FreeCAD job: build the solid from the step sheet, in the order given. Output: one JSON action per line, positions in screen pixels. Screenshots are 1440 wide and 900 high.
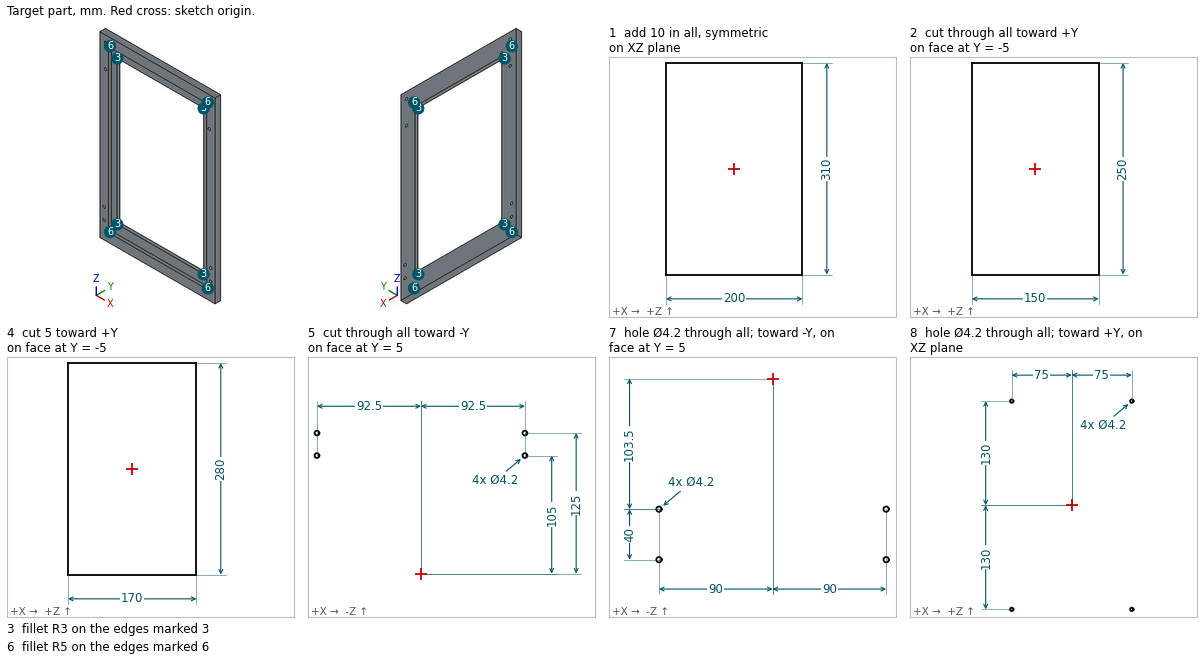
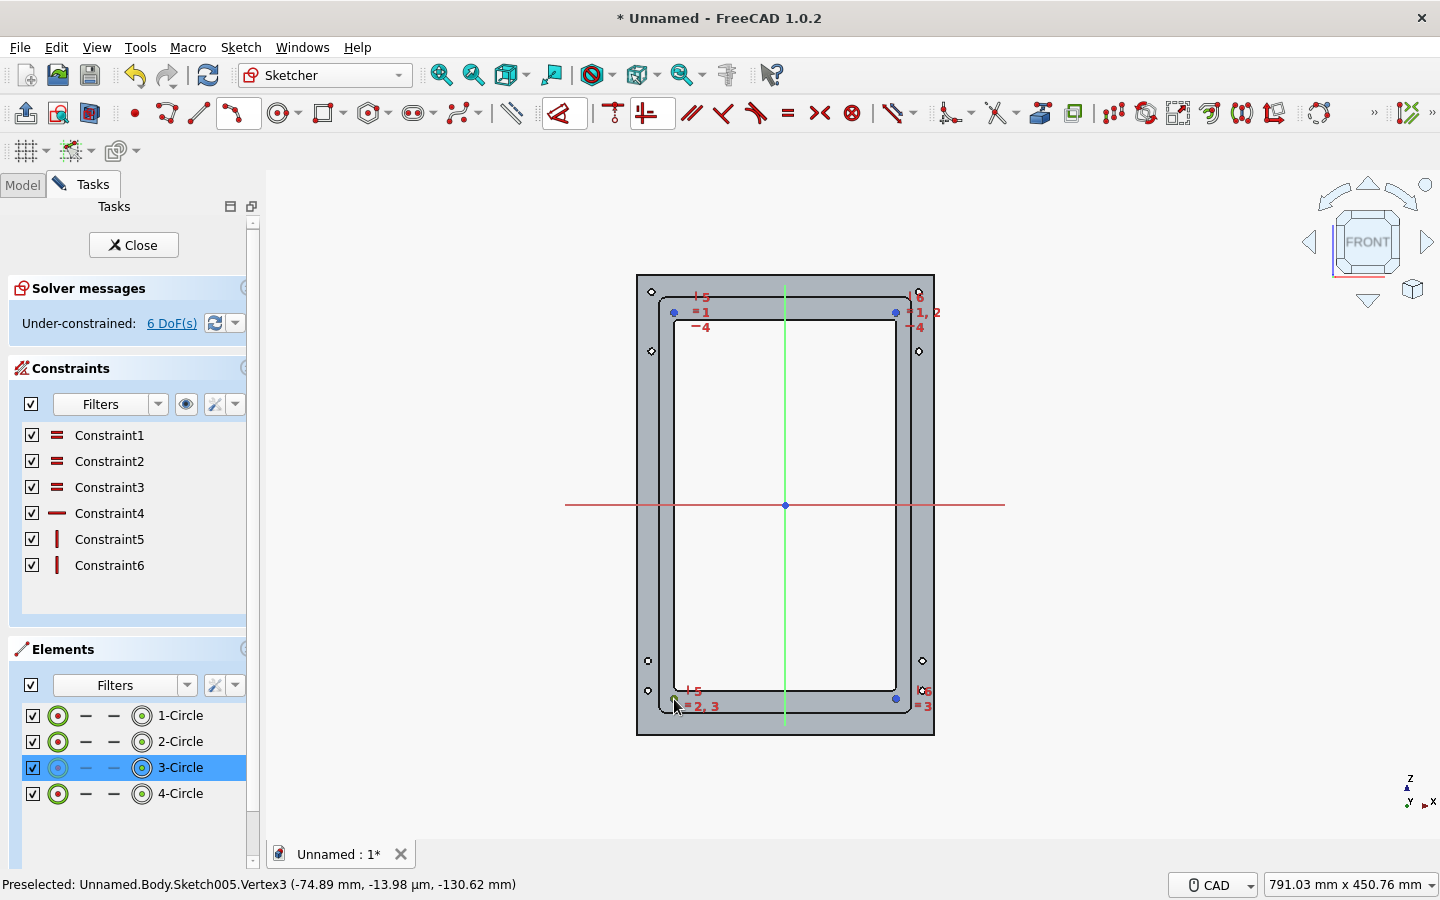
{"action": "left_click", "coordinate": [896, 699]}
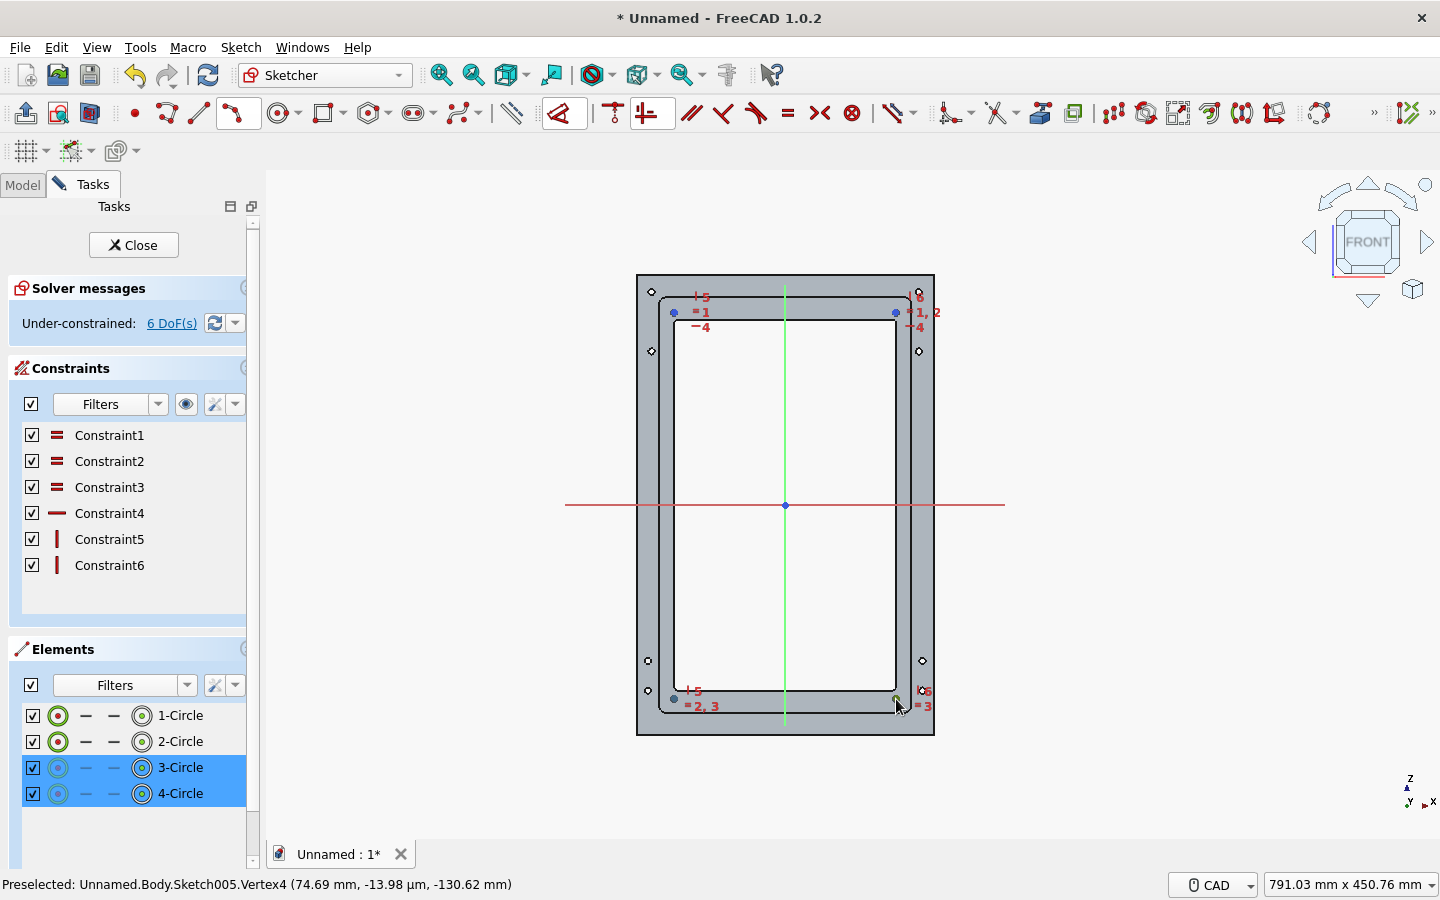
{"action": "key", "text": "h"}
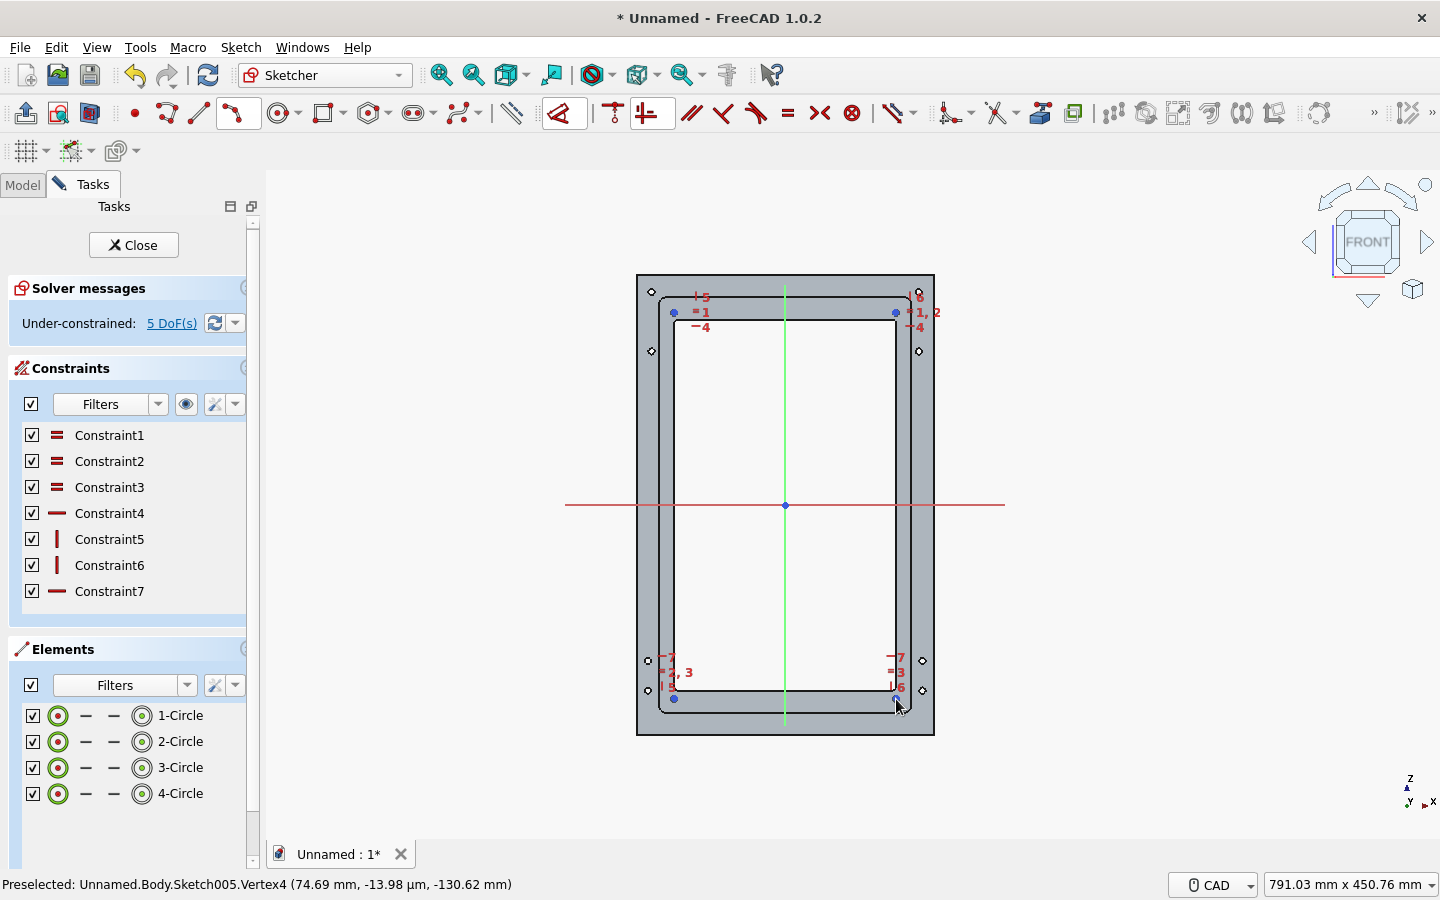
{"action": "scroll", "coordinate": [676, 310], "scroll_direction": "up", "scroll_amount": 10}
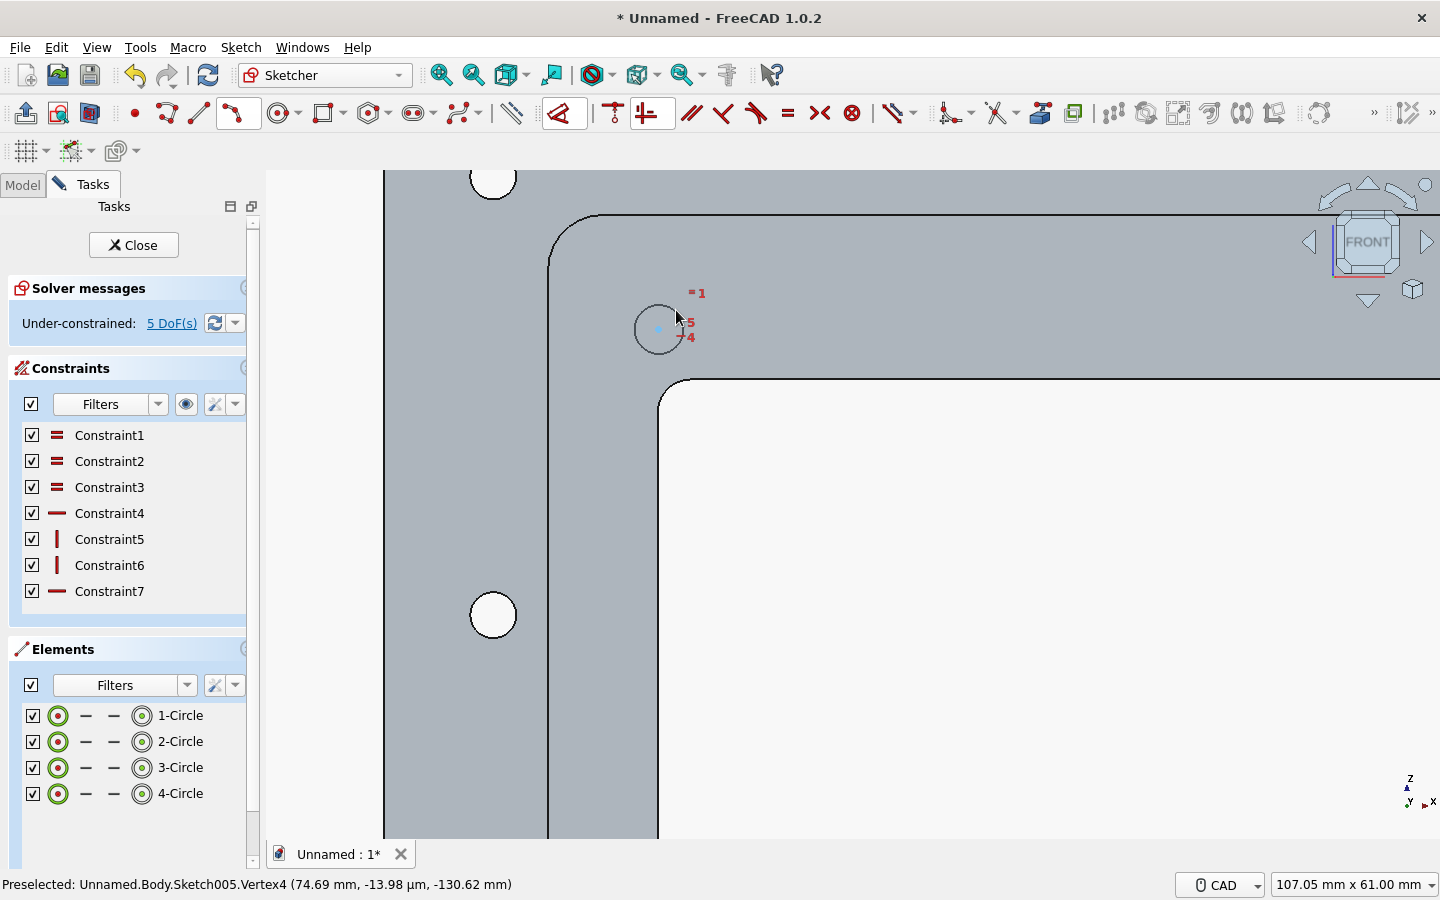
{"action": "left_click", "coordinate": [676, 312]}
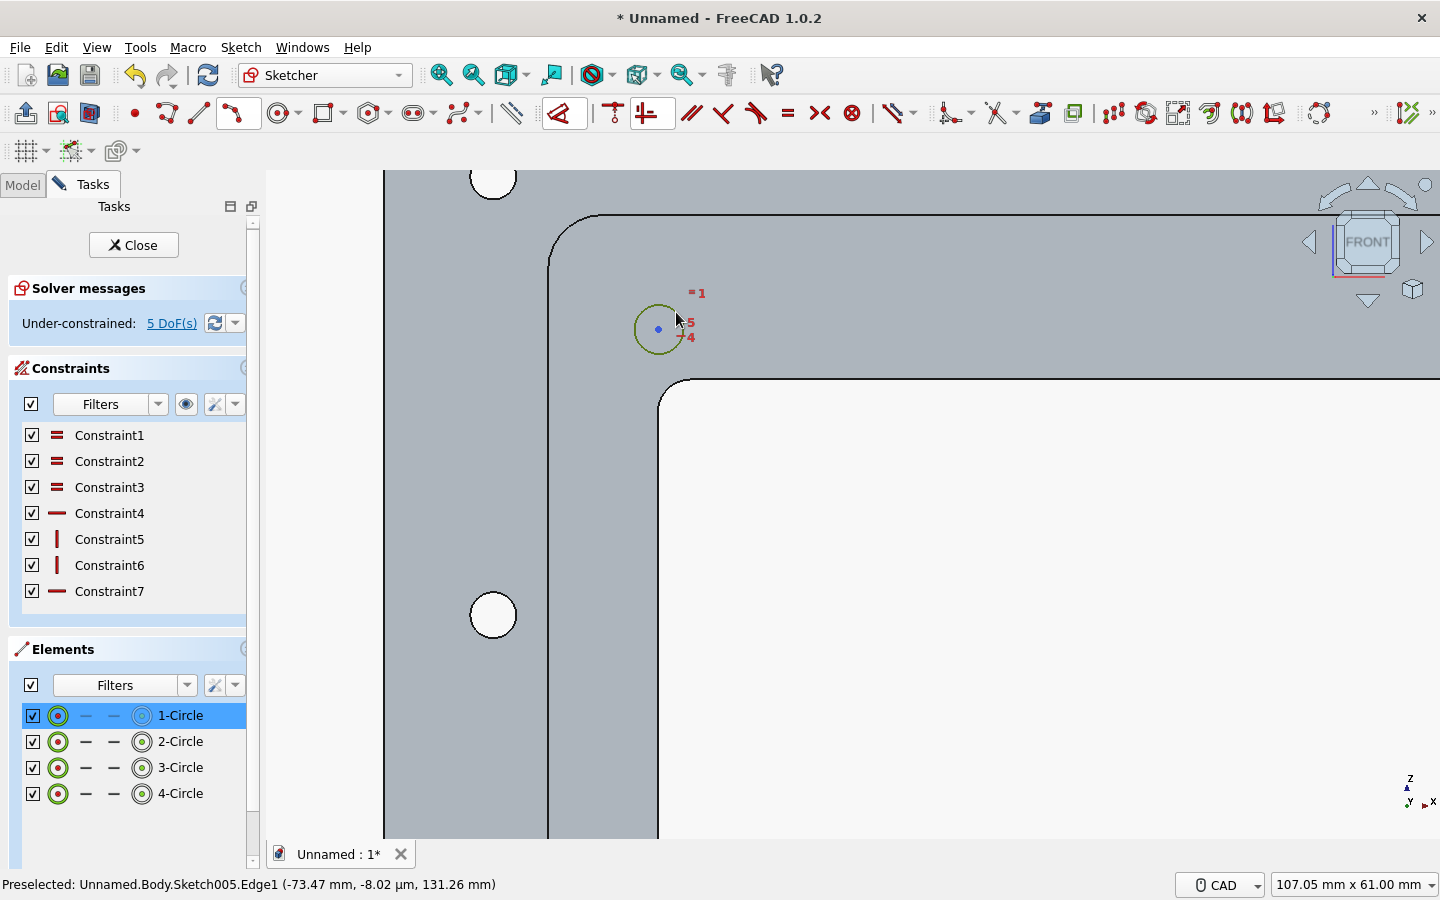
{"action": "key", "text": "k o"}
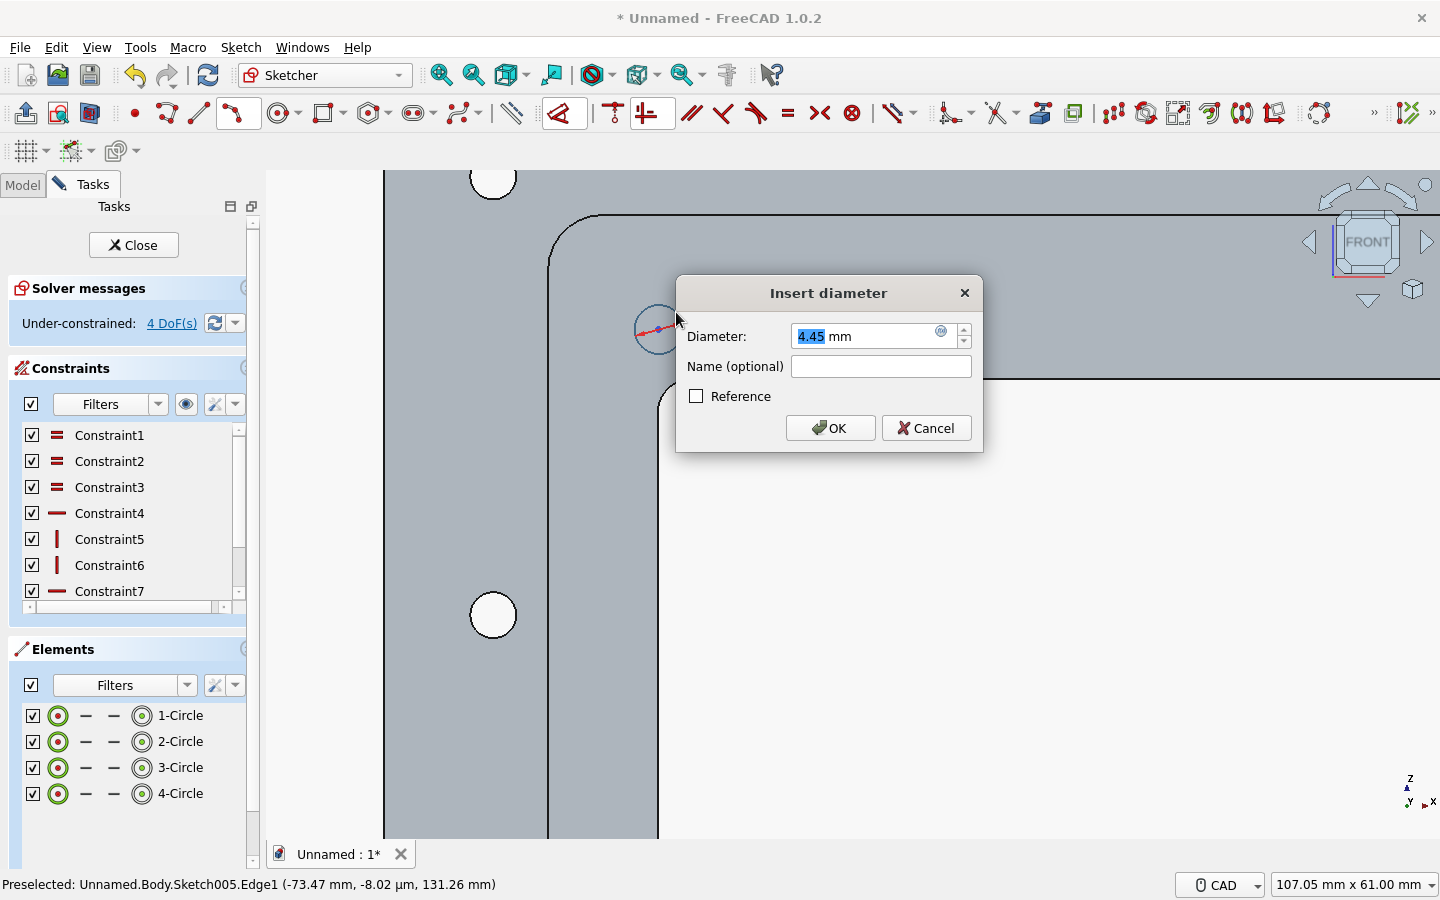
{"action": "type", "text": "4.2"}
{"action": "key", "text": "Return"}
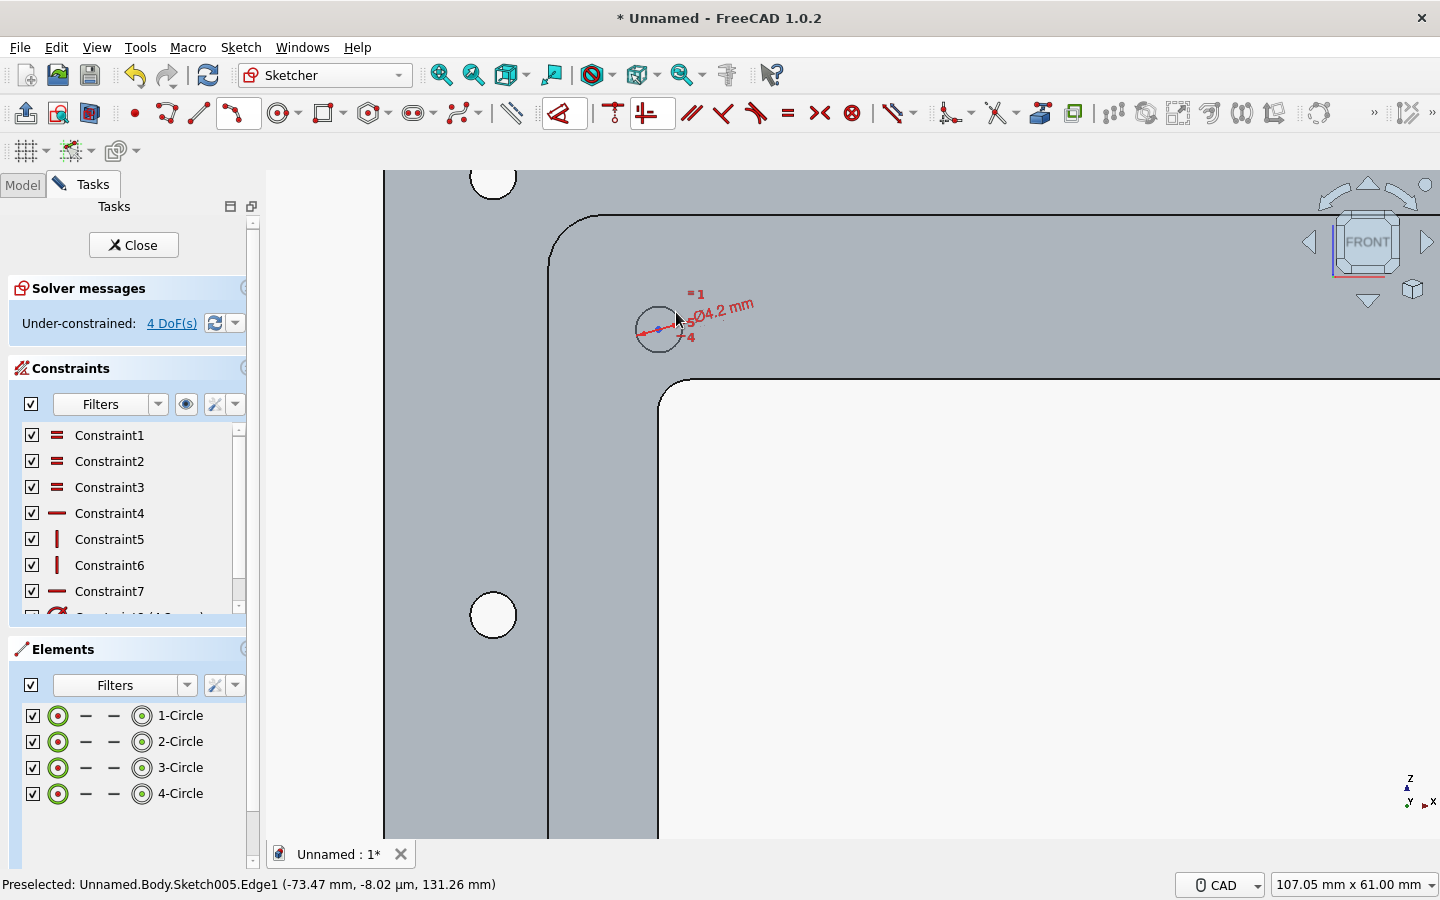
{"action": "scroll", "coordinate": [676, 310], "scroll_direction": "down", "scroll_amount": 10}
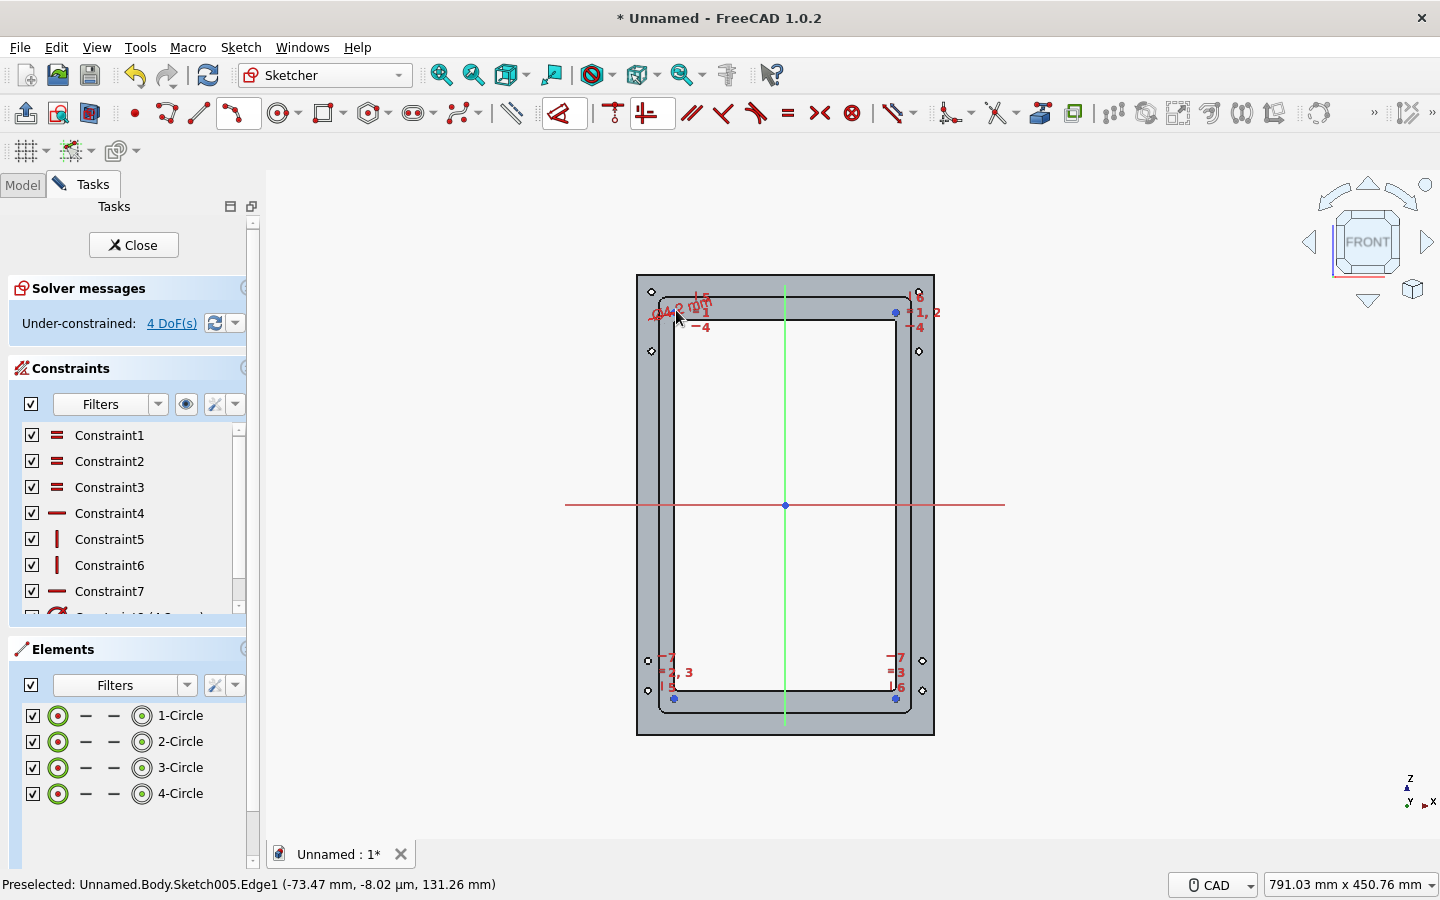
{"action": "left_click", "coordinate": [674, 313]}